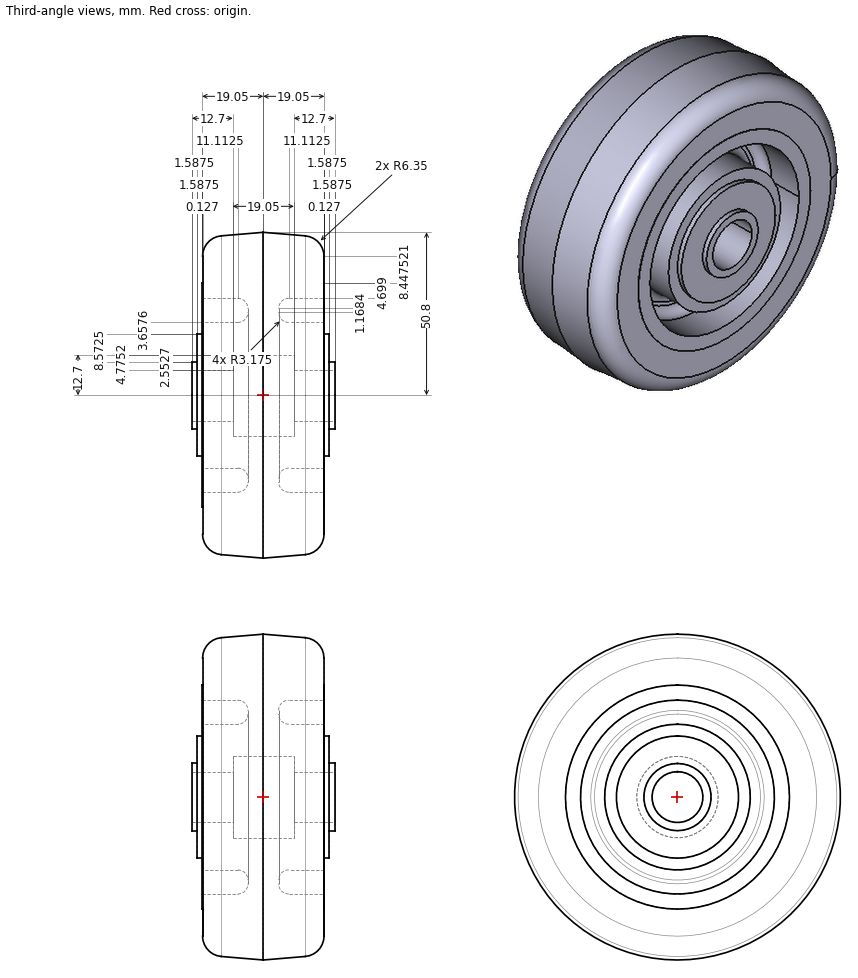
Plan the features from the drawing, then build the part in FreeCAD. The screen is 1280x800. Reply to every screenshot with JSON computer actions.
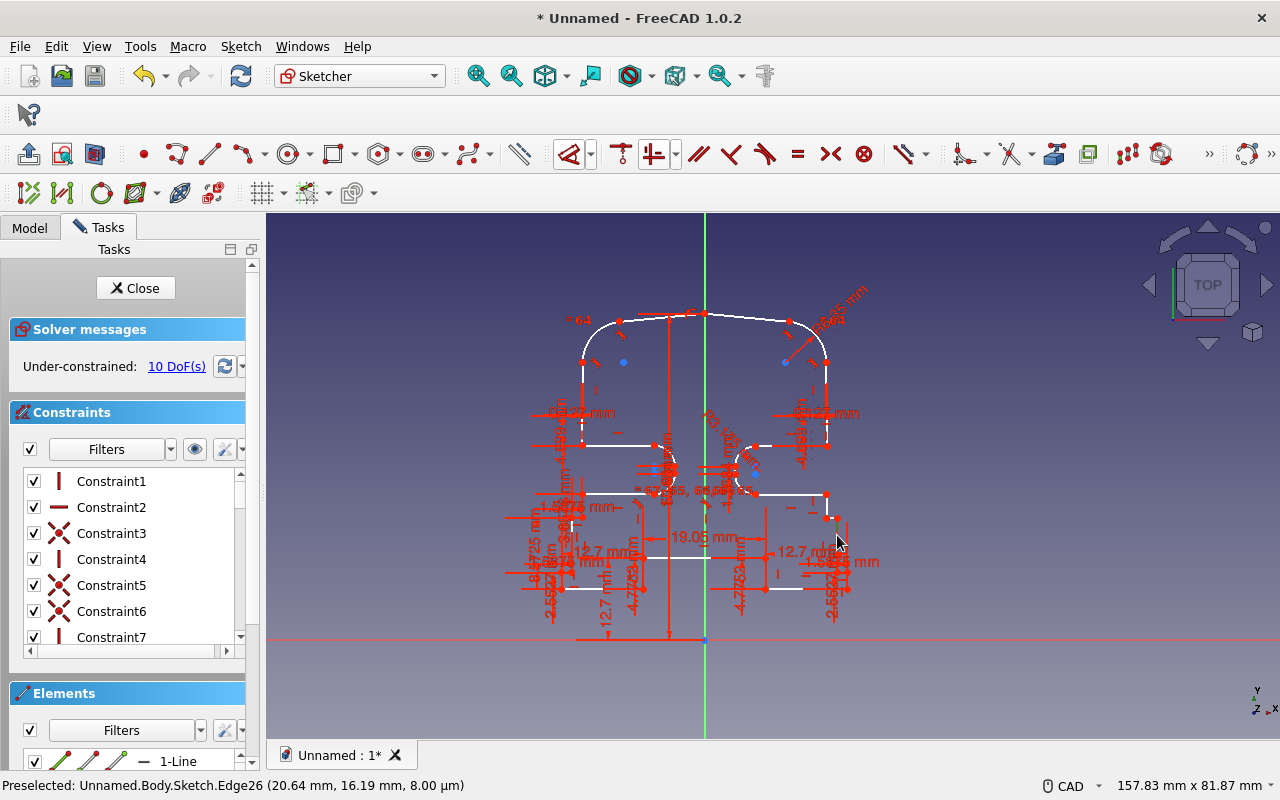
{"action": "left_click", "coordinate": [590, 154]}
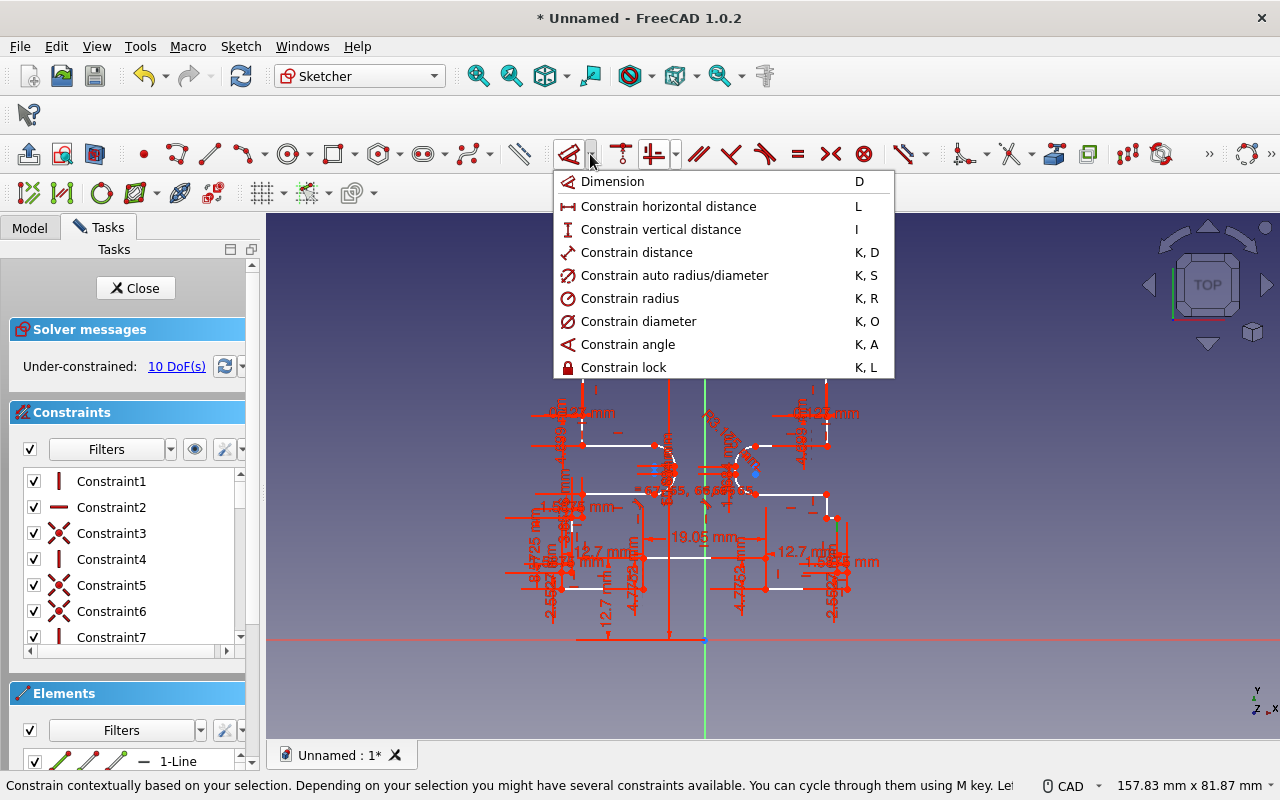
{"action": "left_click", "coordinate": [724, 230]}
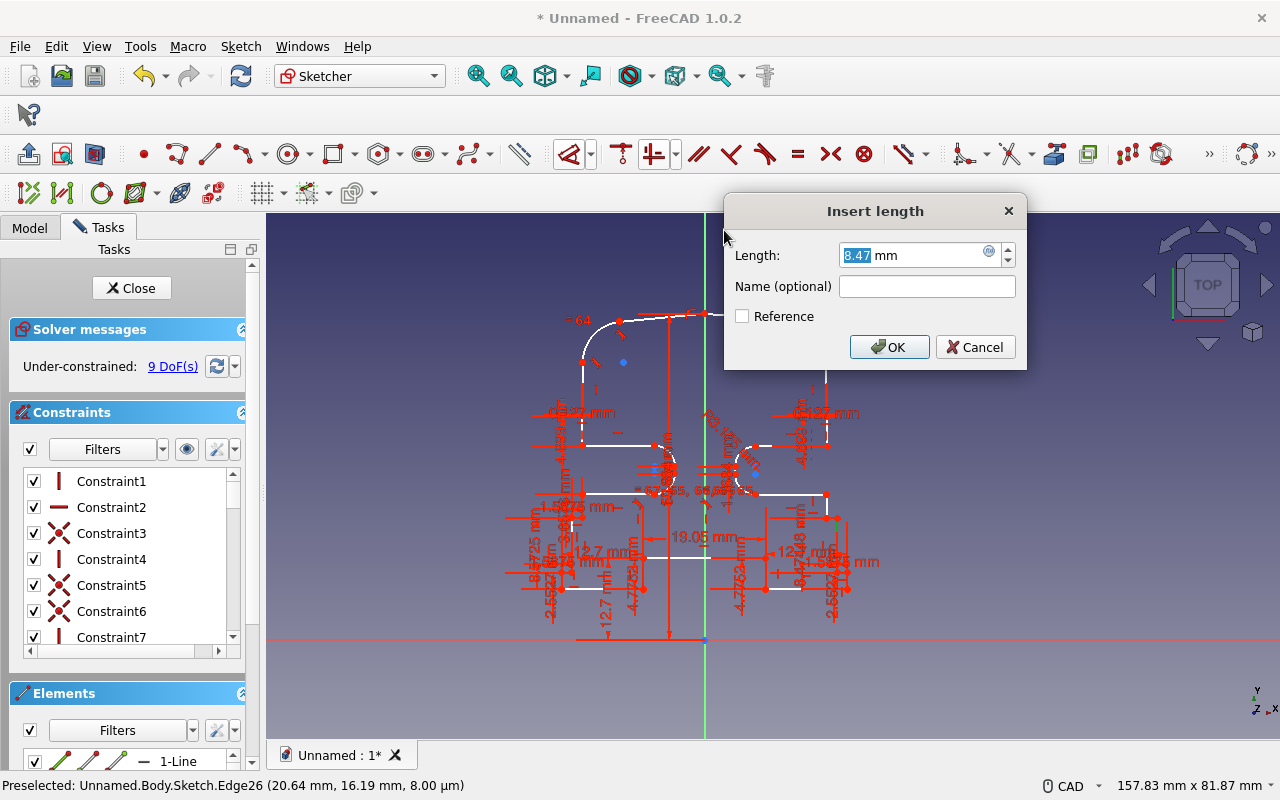
{"action": "type", "text": "8.5725"}
{"action": "key", "text": "Return"}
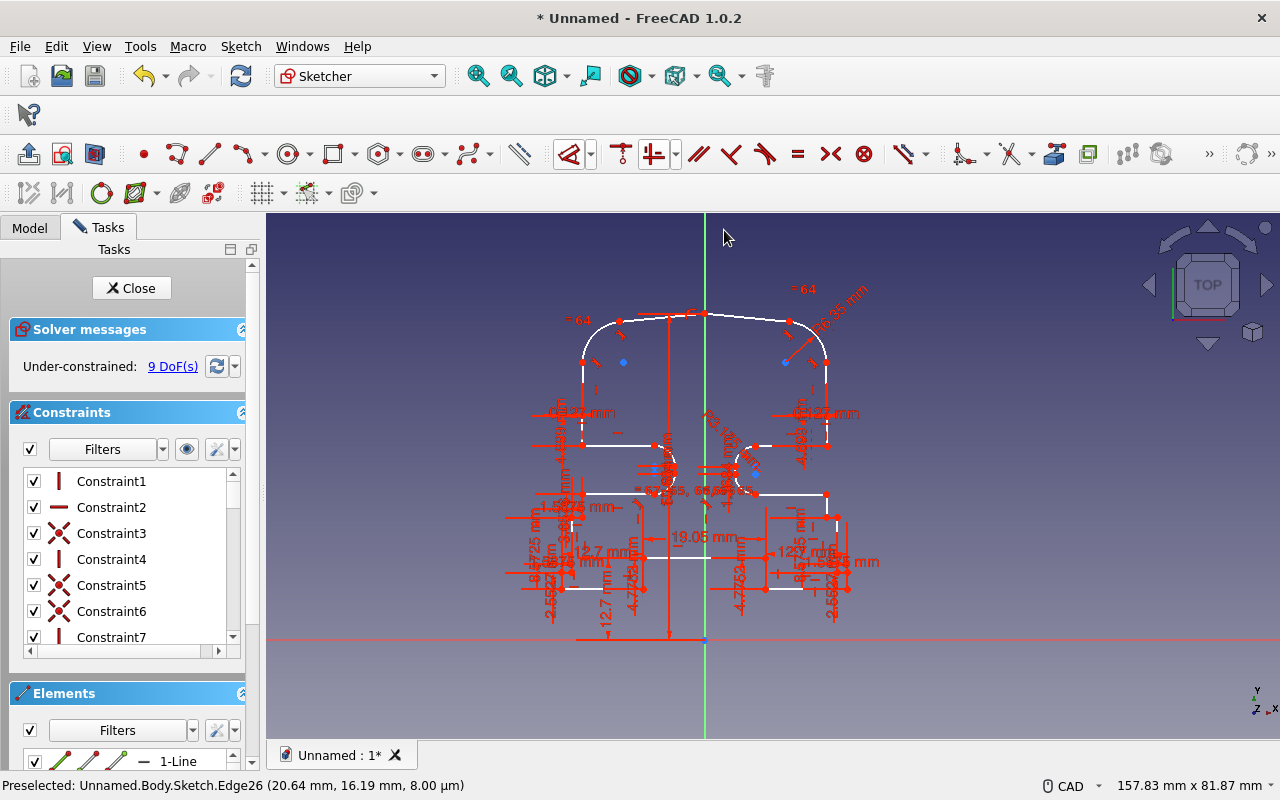
{"action": "scroll", "coordinate": [832, 518], "scroll_direction": "up", "scroll_amount": 7}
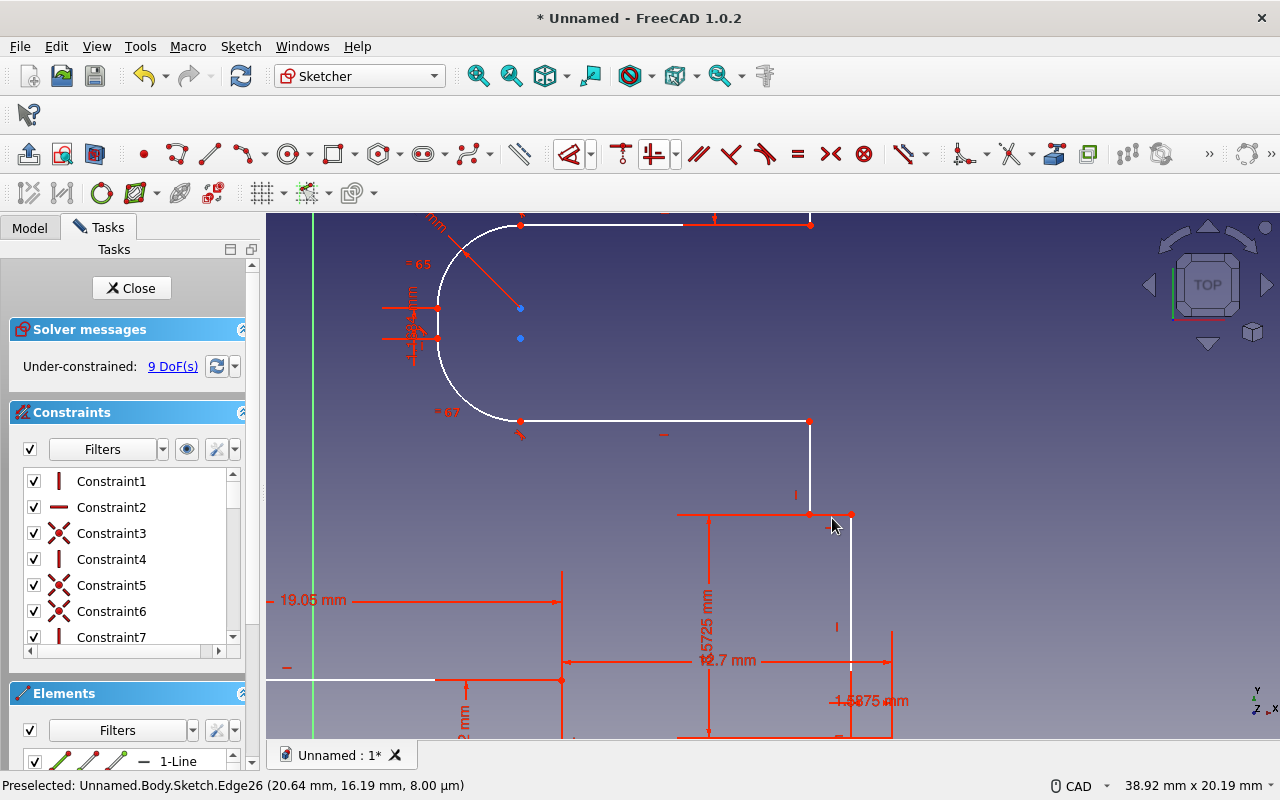
{"action": "left_click", "coordinate": [830, 515]}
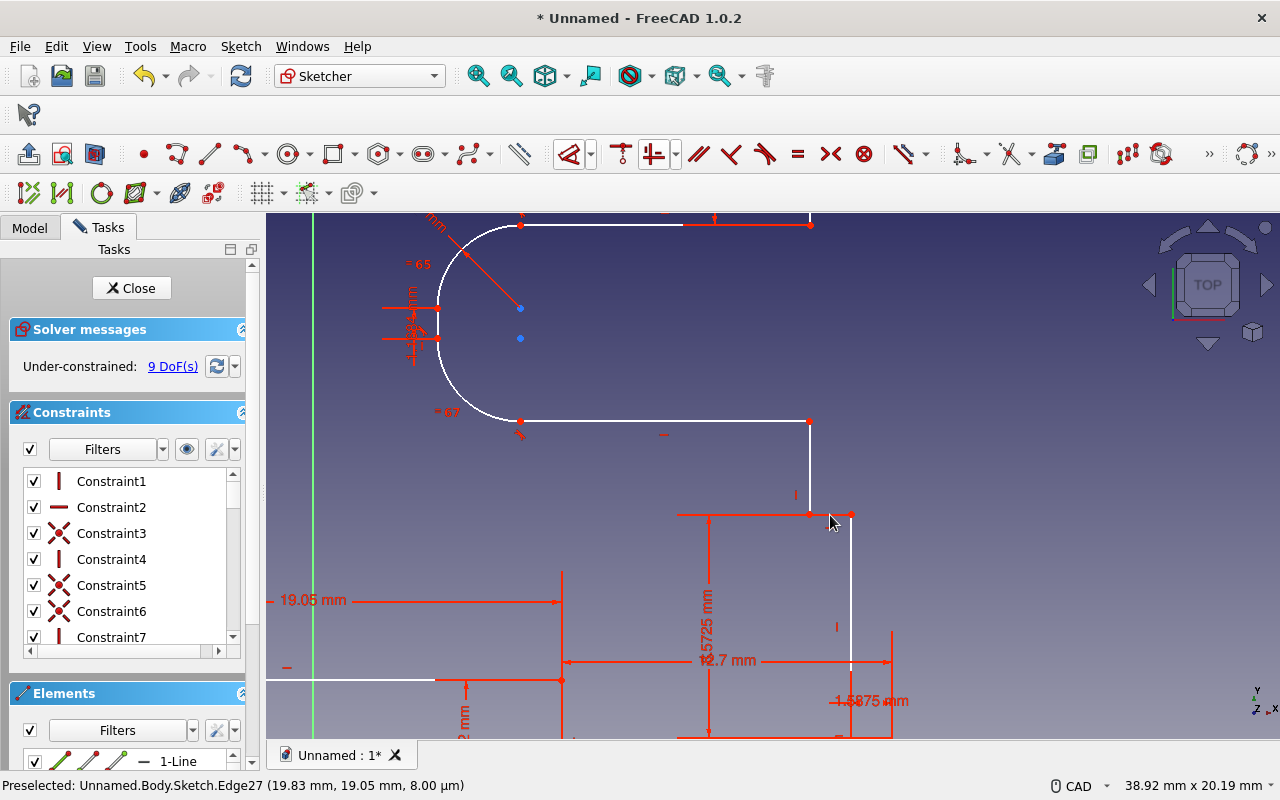
{"action": "key", "text": "l"}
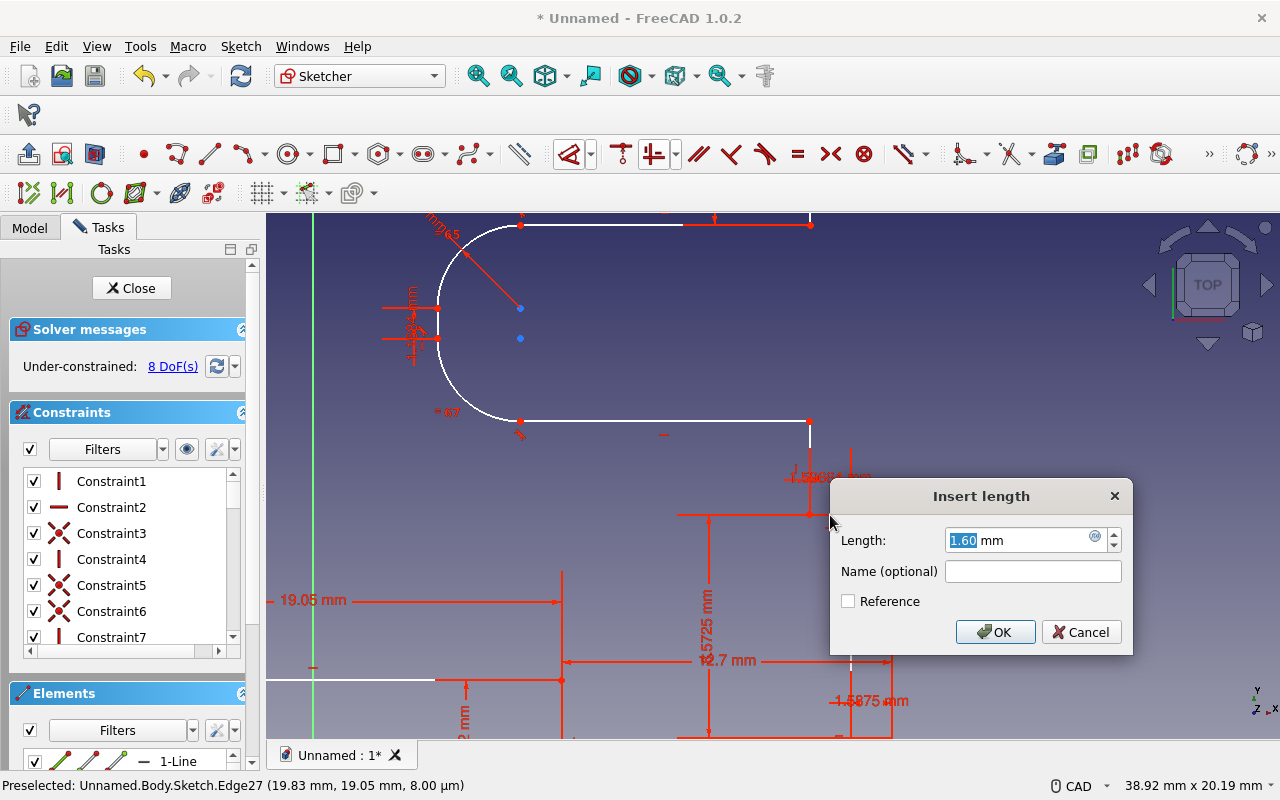
{"action": "type", "text": "1.5875"}
{"action": "key", "text": "Return"}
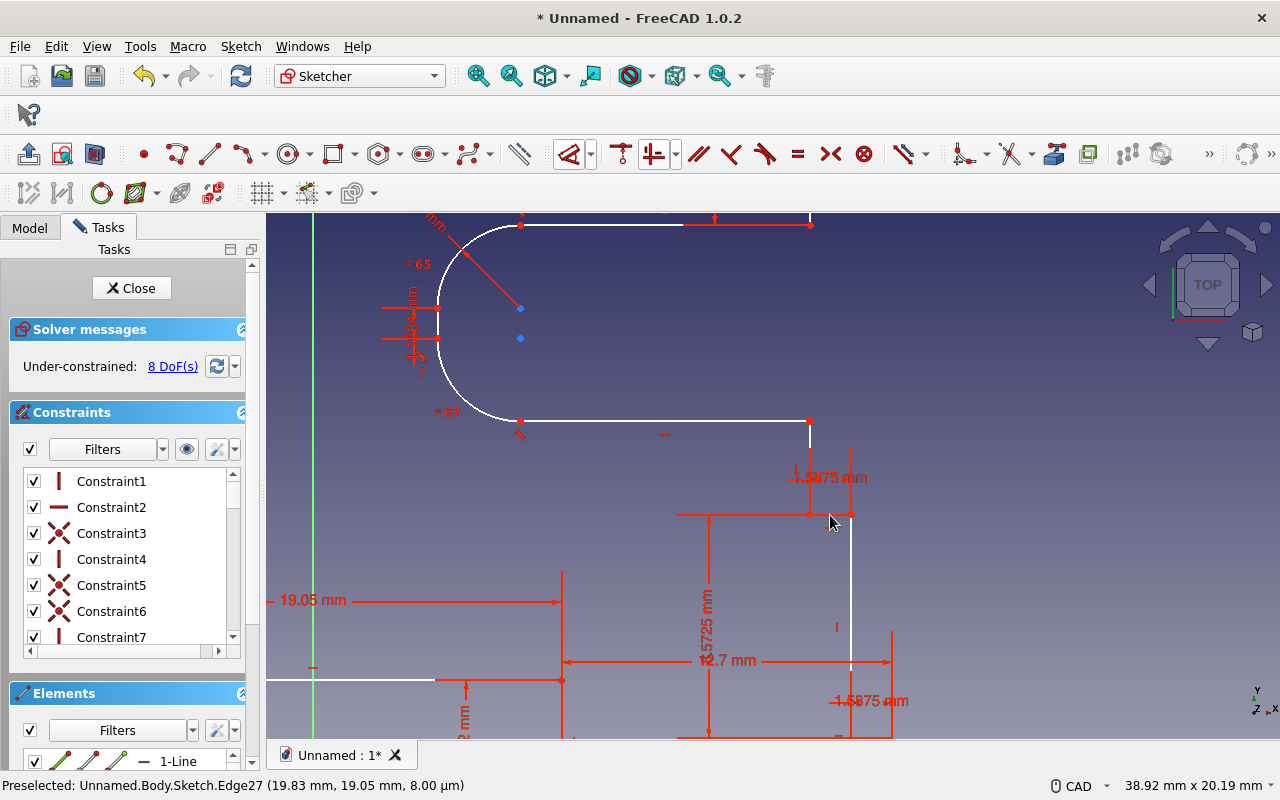
{"action": "left_click", "coordinate": [810, 487]}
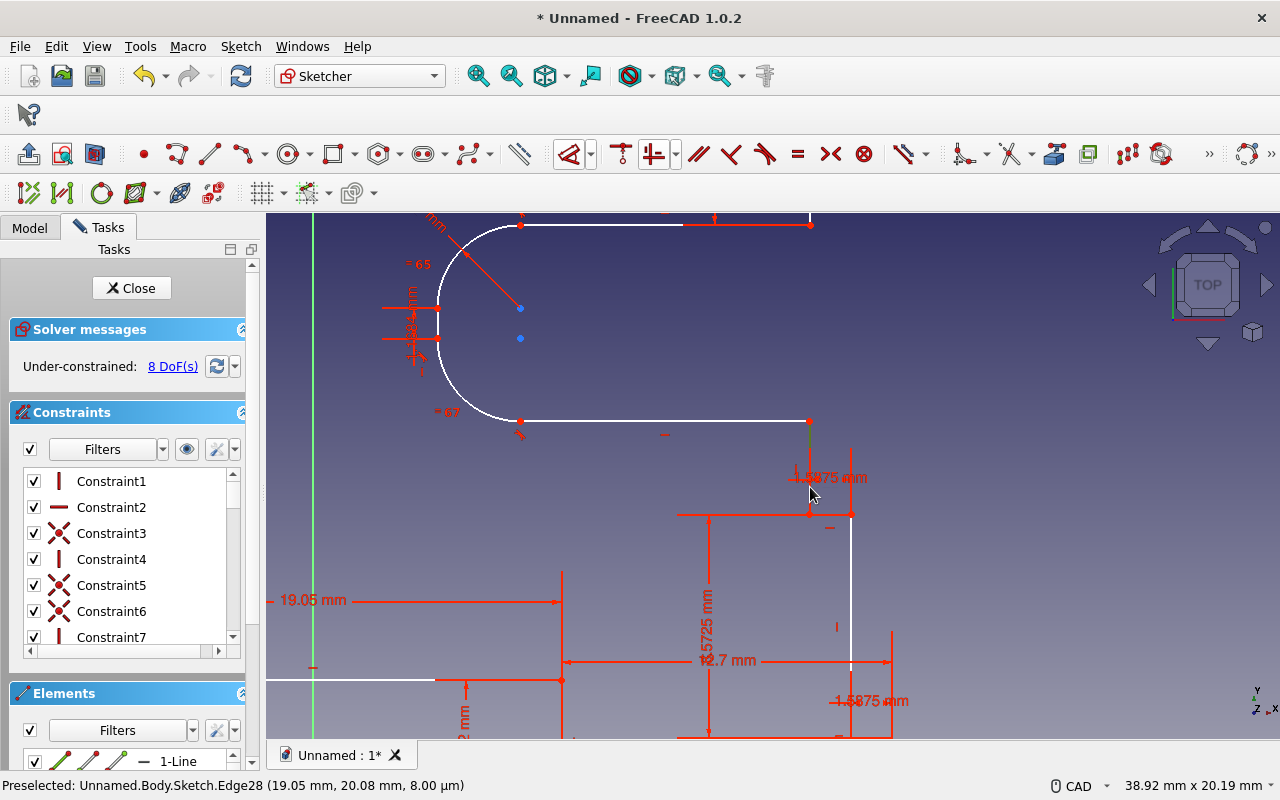
{"action": "key", "text": "i"}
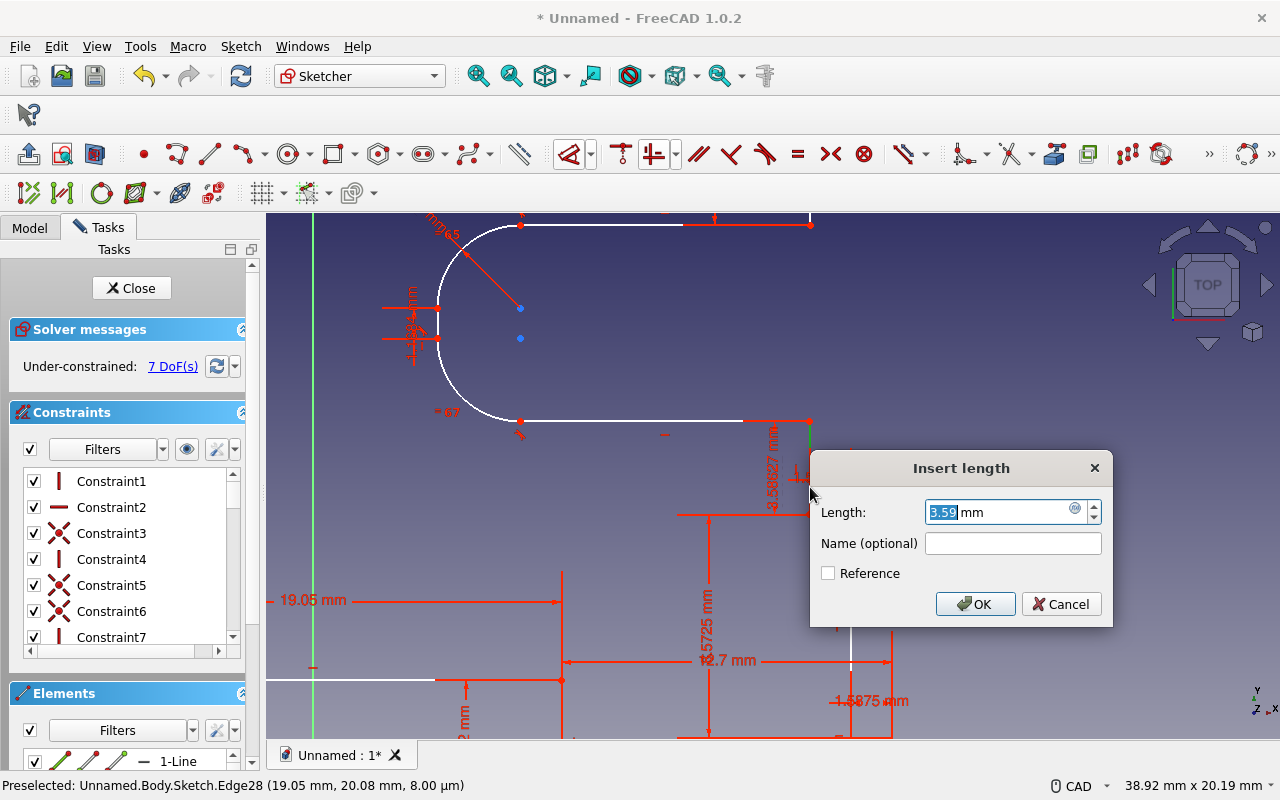
{"action": "type", "text": "3.6576"}
{"action": "key", "text": "Return"}